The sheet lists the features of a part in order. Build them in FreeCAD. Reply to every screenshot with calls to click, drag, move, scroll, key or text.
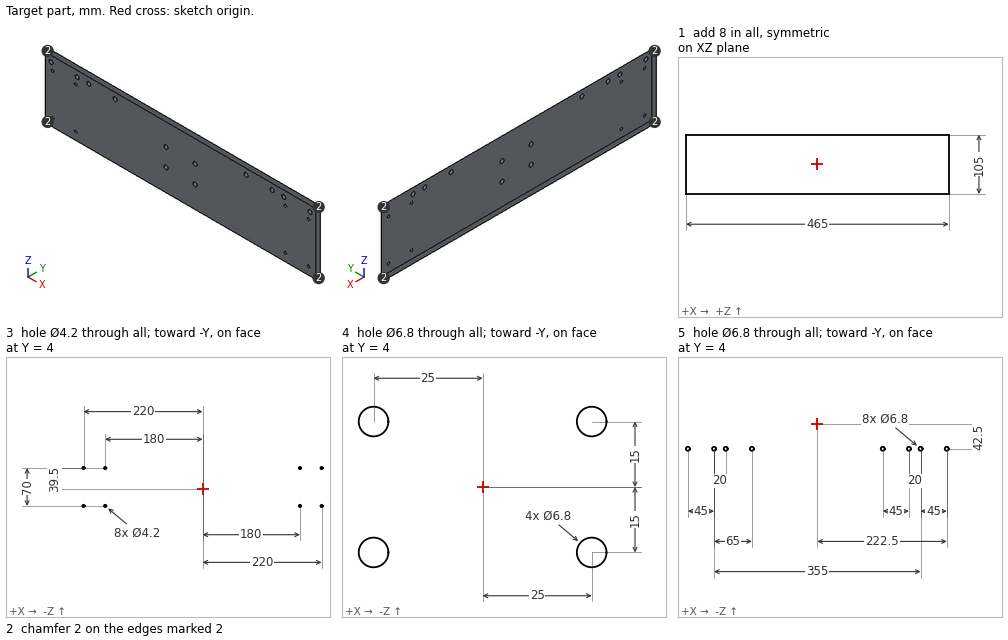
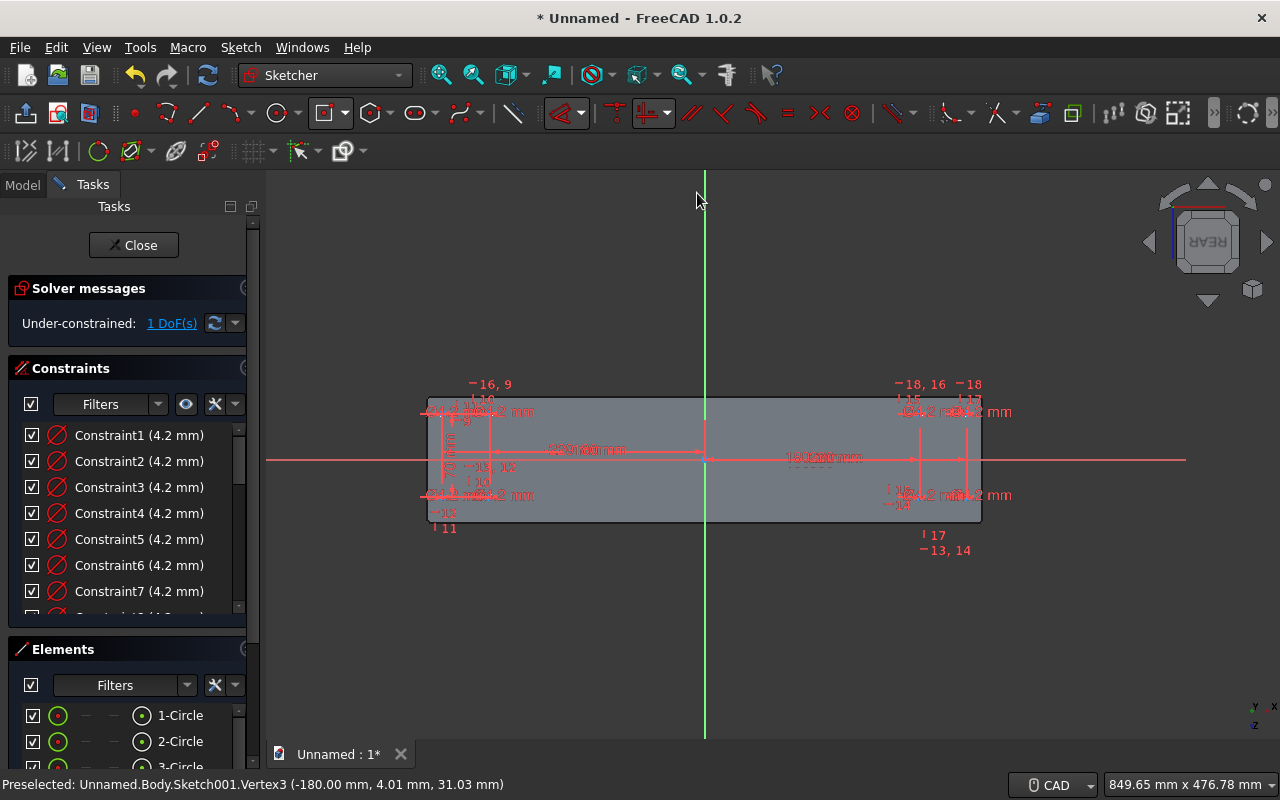
click(442, 414)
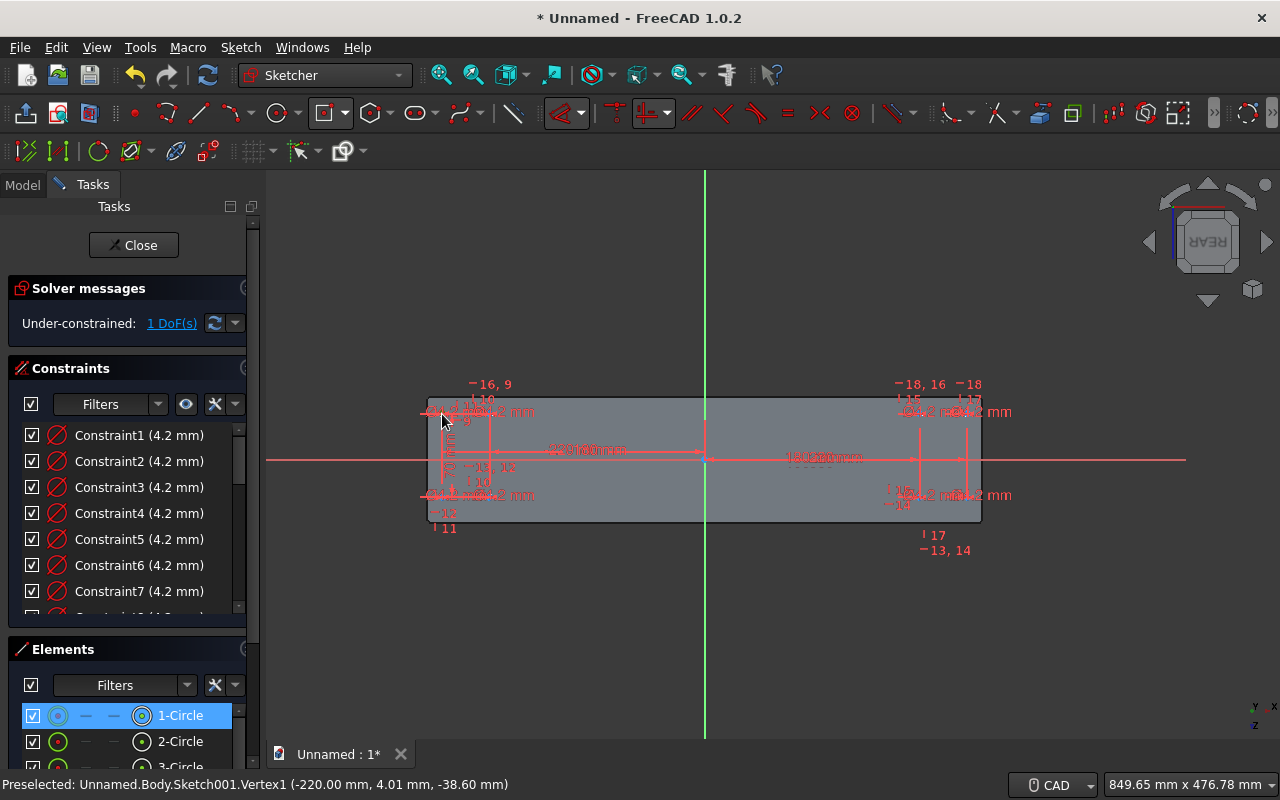
click(584, 114)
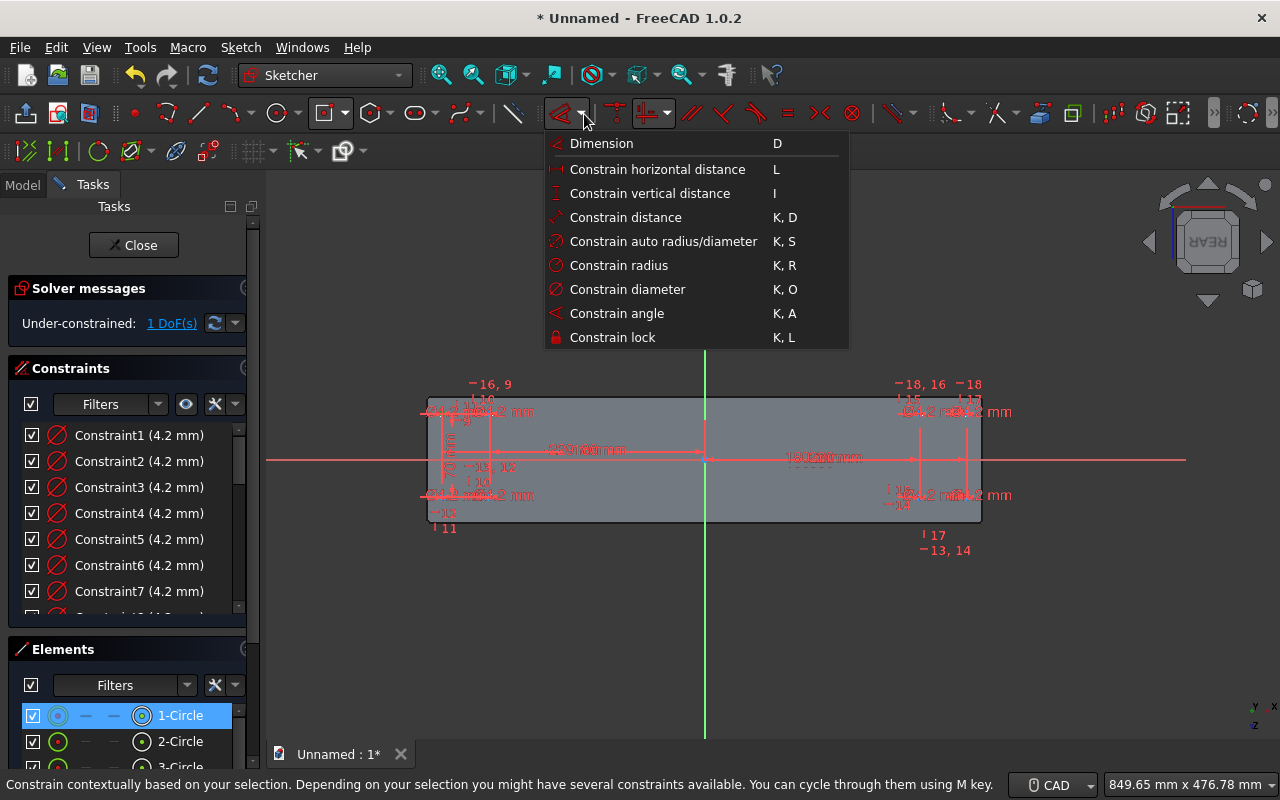
click(697, 193)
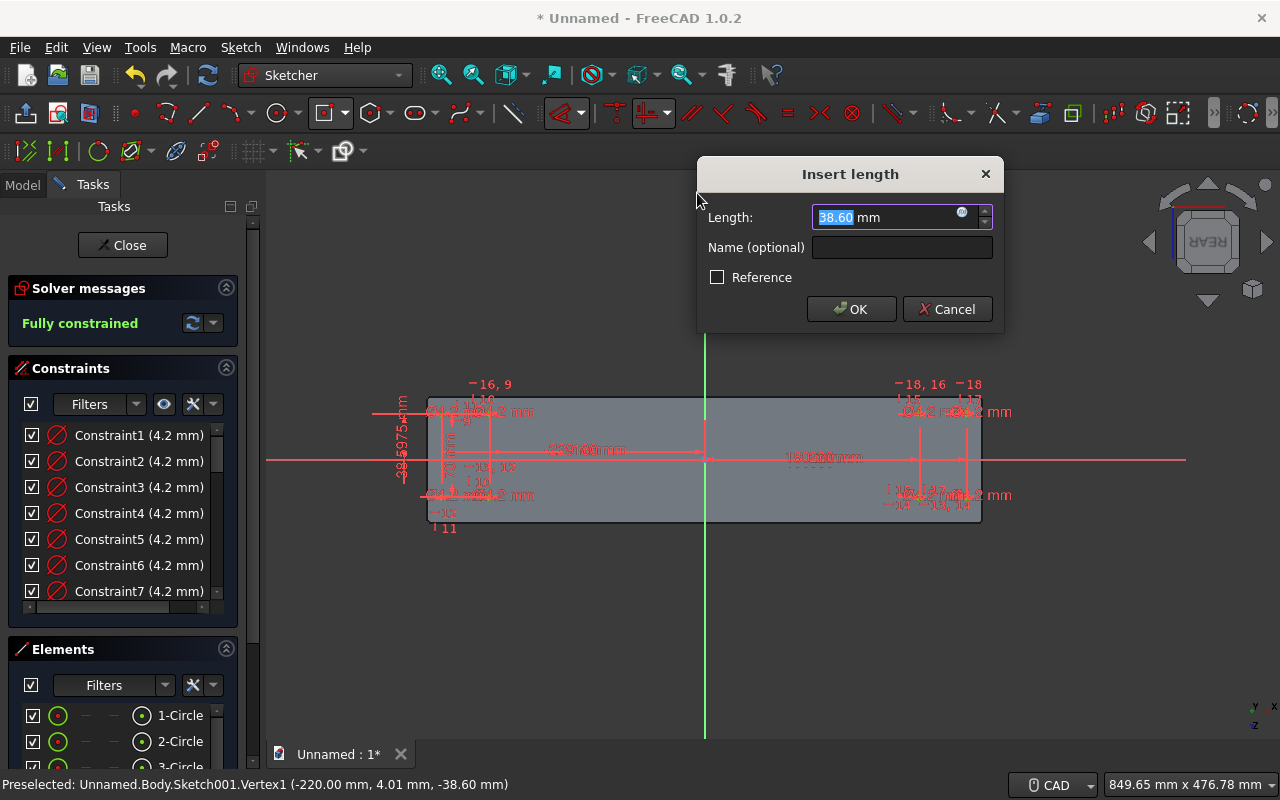
text(39.5)
key(Return)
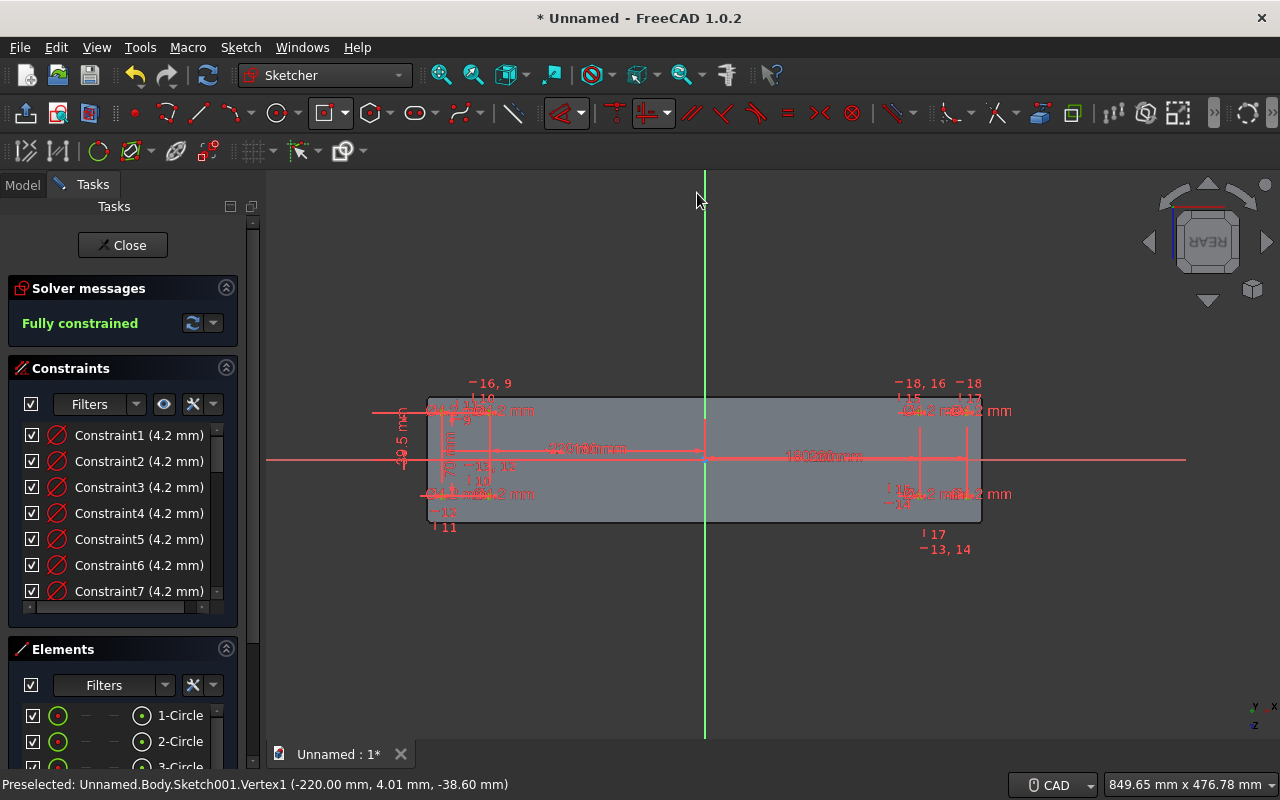
click(123, 245)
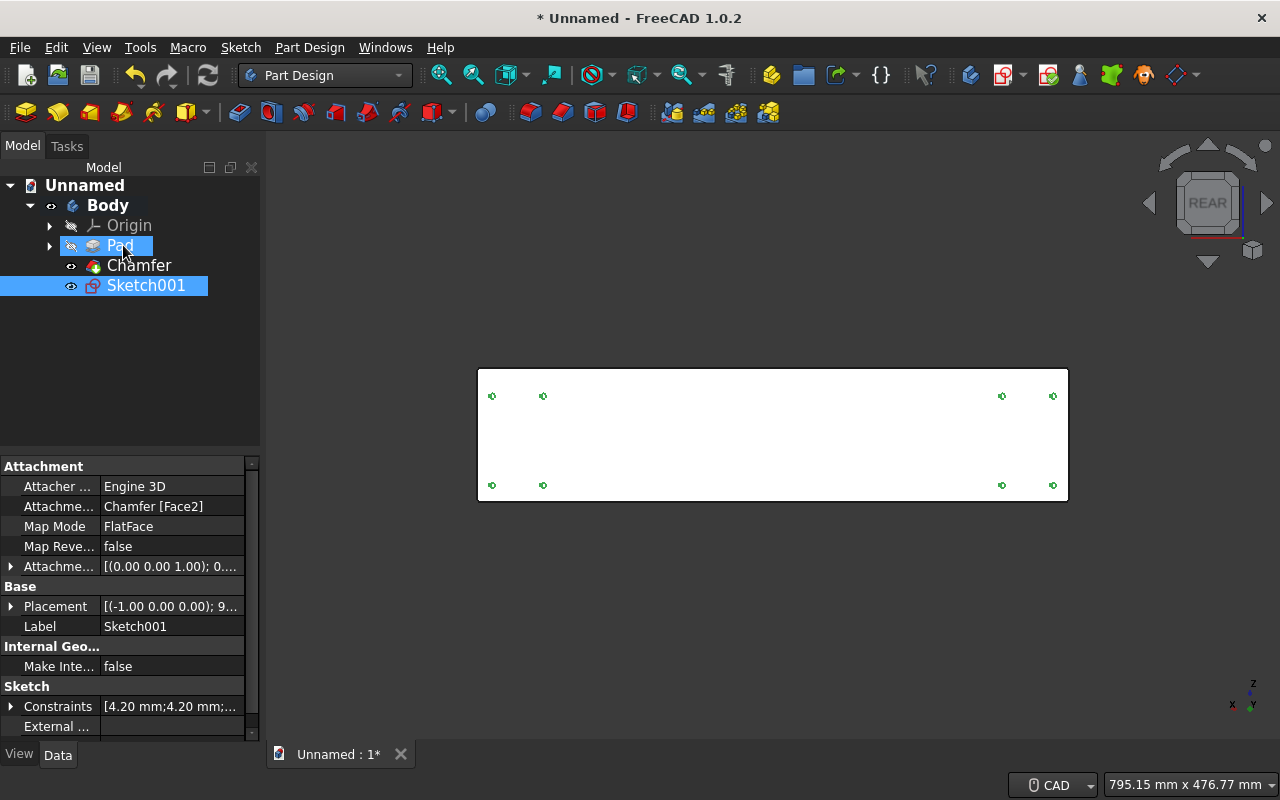
click(272, 112)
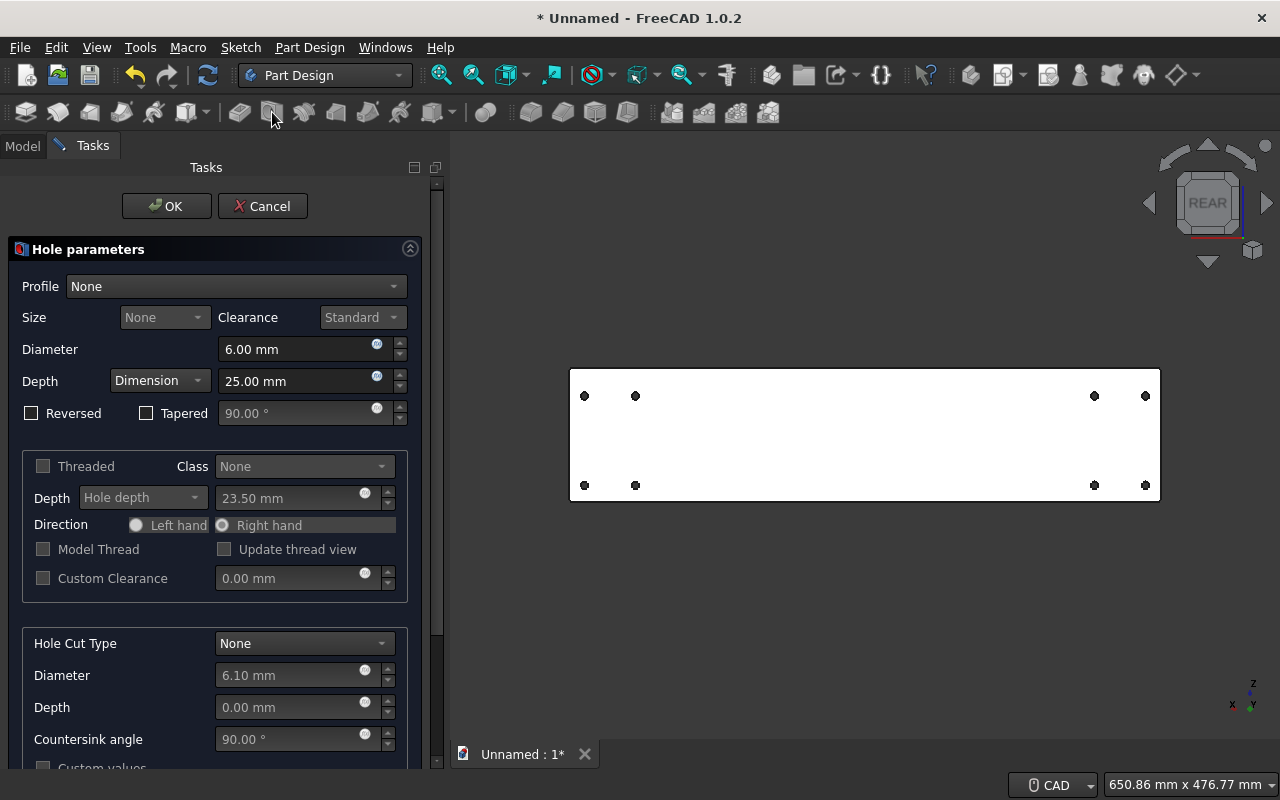
triple_click(305, 349)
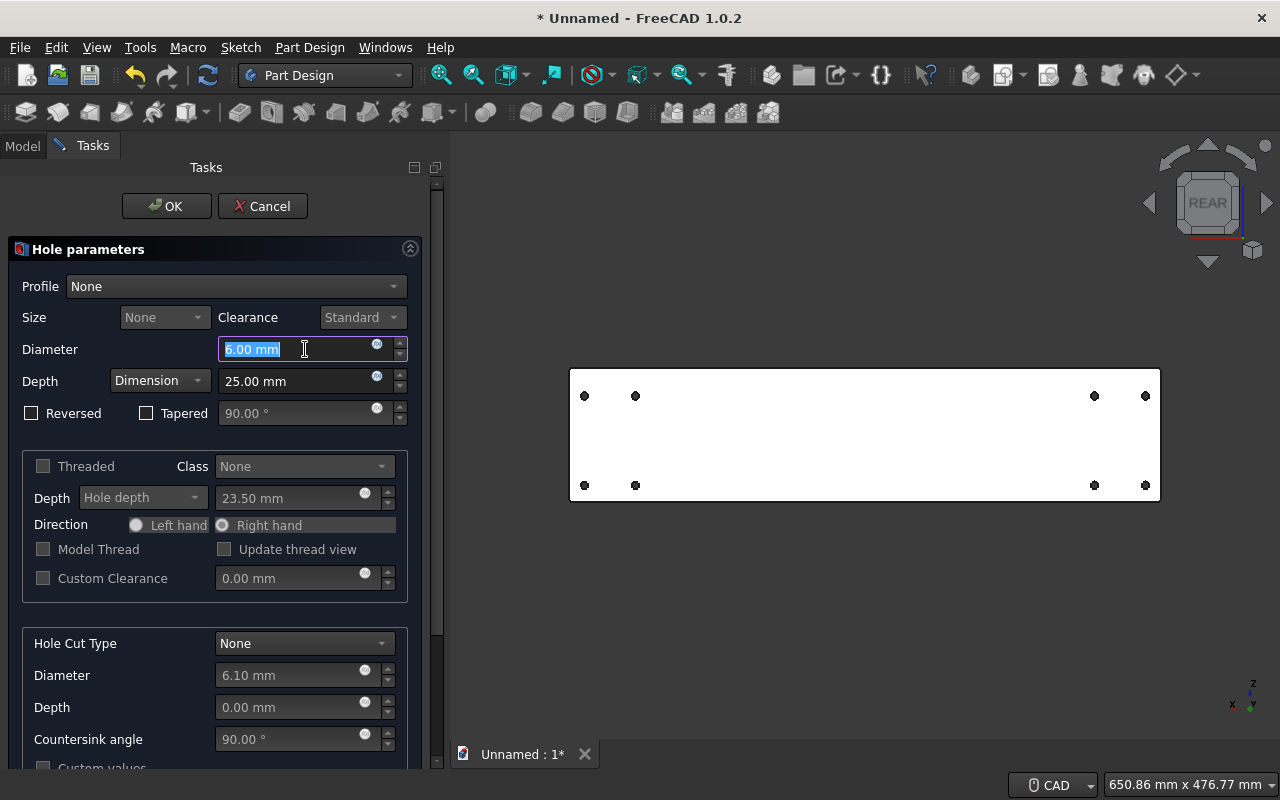
text(4.2)
key(Tab)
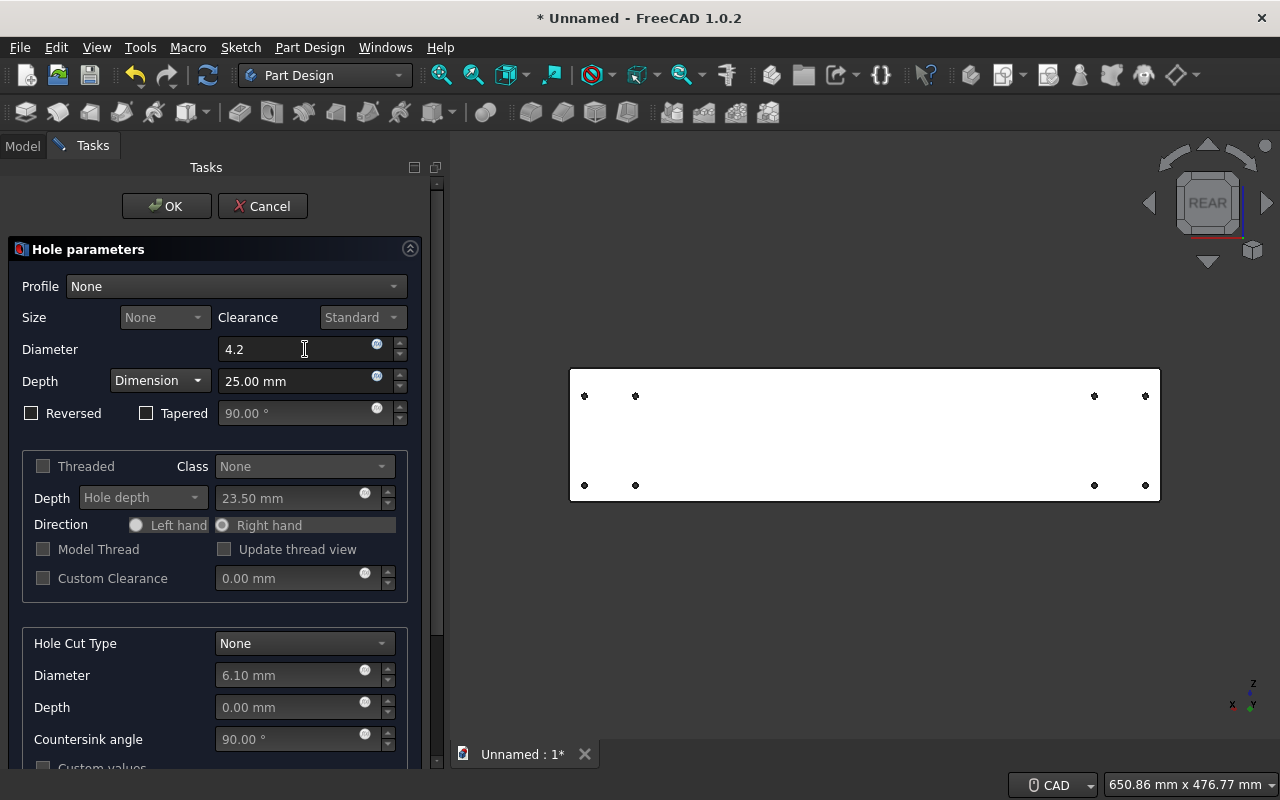
click(161, 380)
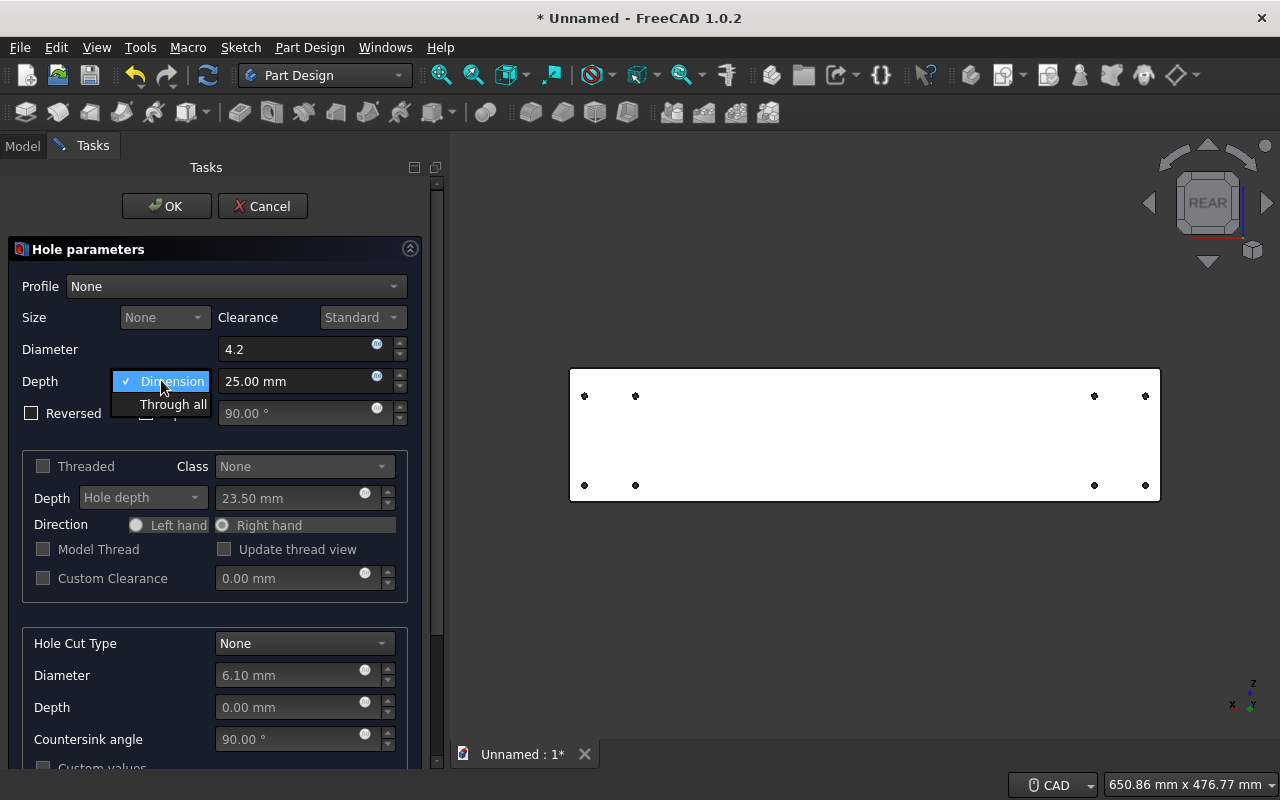
click(160, 404)